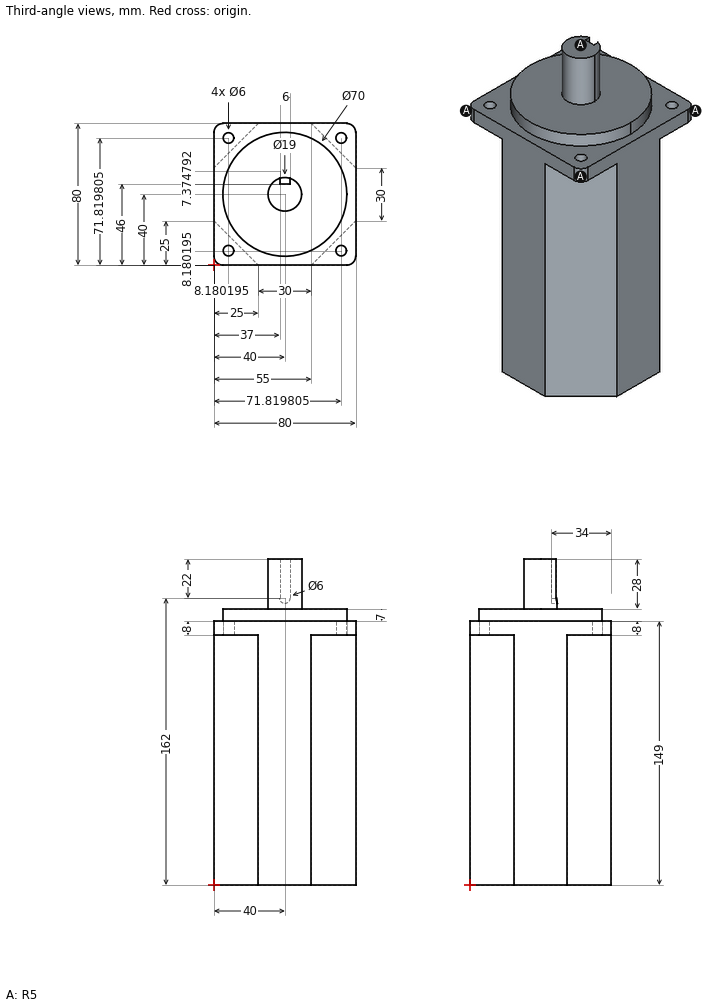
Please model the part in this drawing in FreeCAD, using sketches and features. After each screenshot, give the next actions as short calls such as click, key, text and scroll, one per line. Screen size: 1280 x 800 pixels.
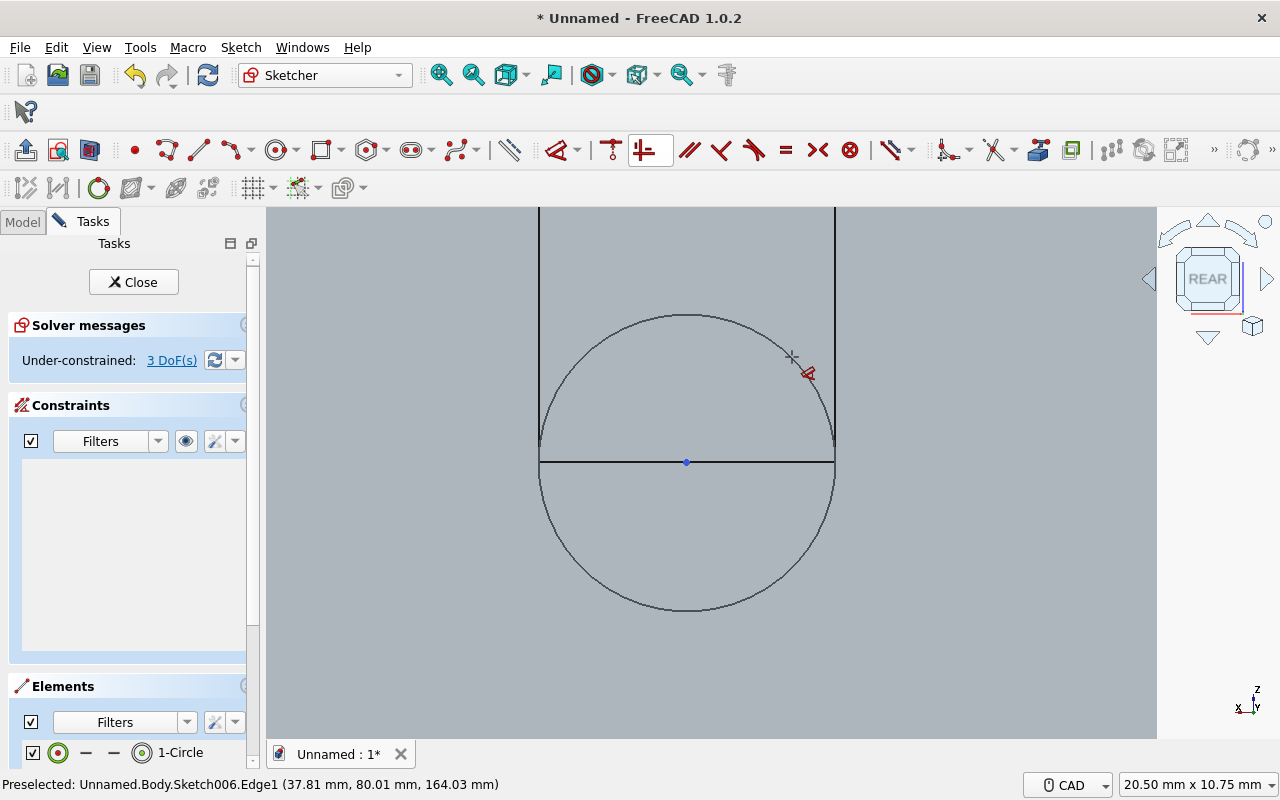
click(792, 358)
click(815, 335)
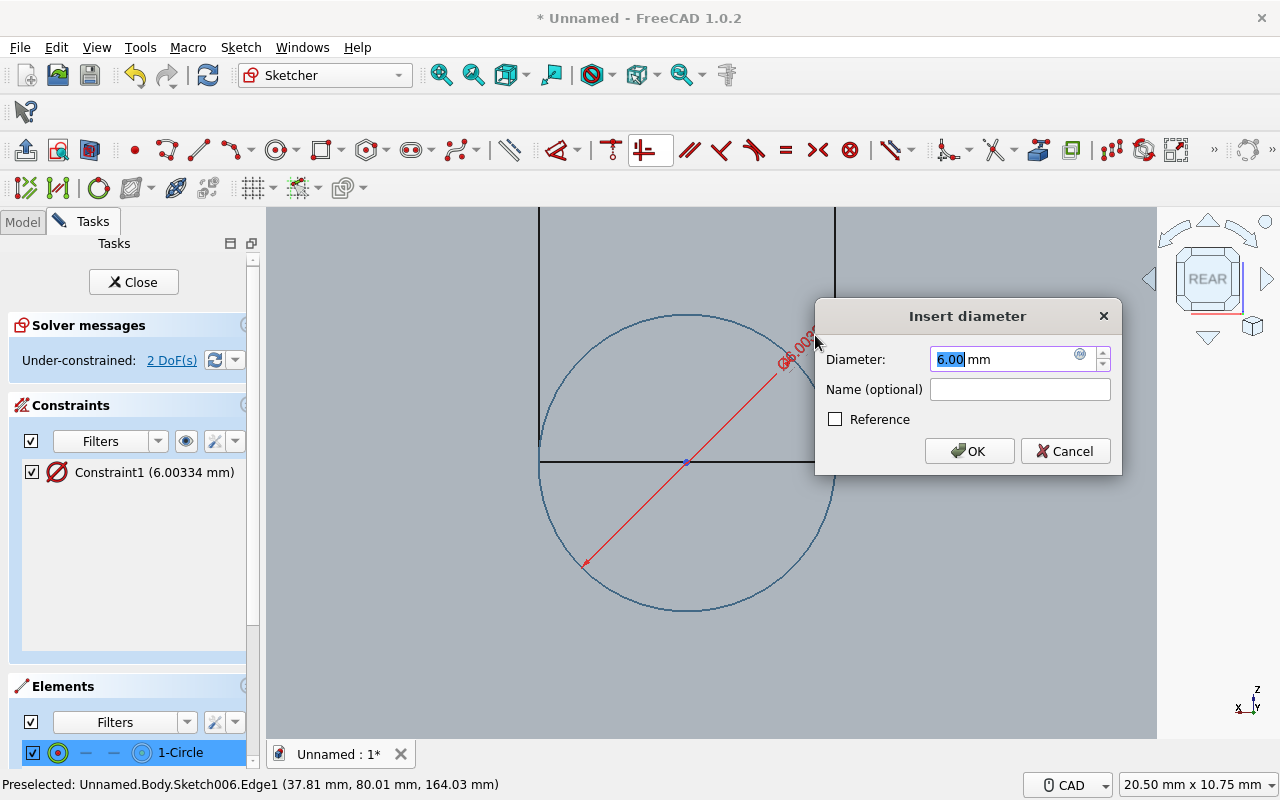
text(6)
key(Return)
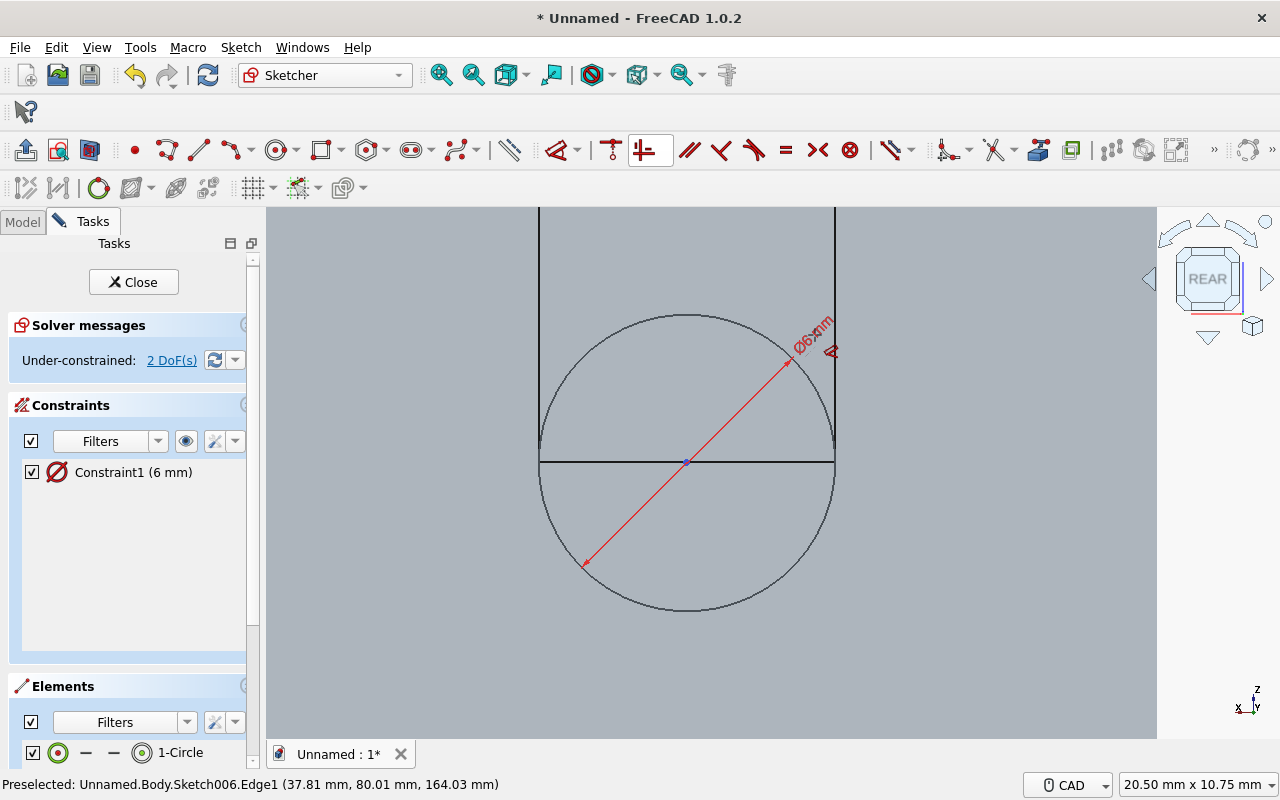
click(687, 463)
click(901, 429)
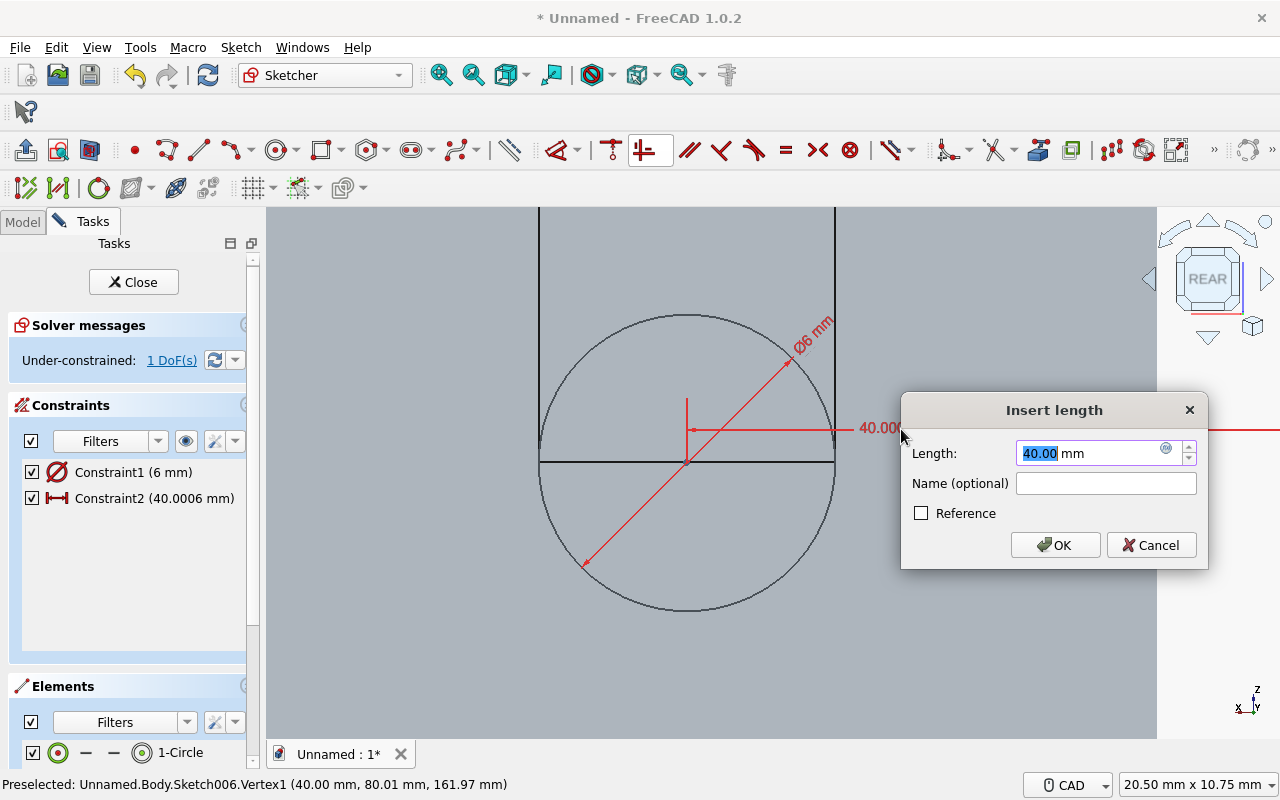
text(40)
key(Return)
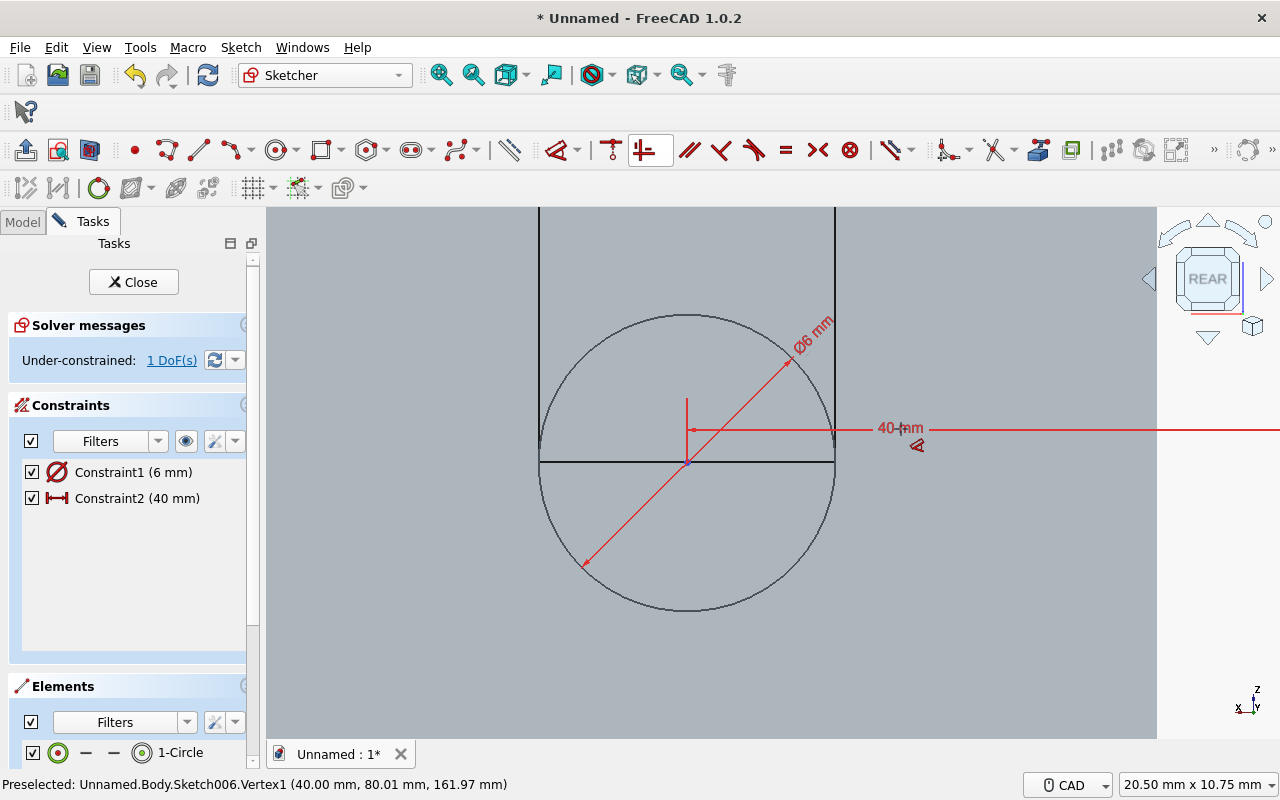
click(687, 463)
click(653, 587)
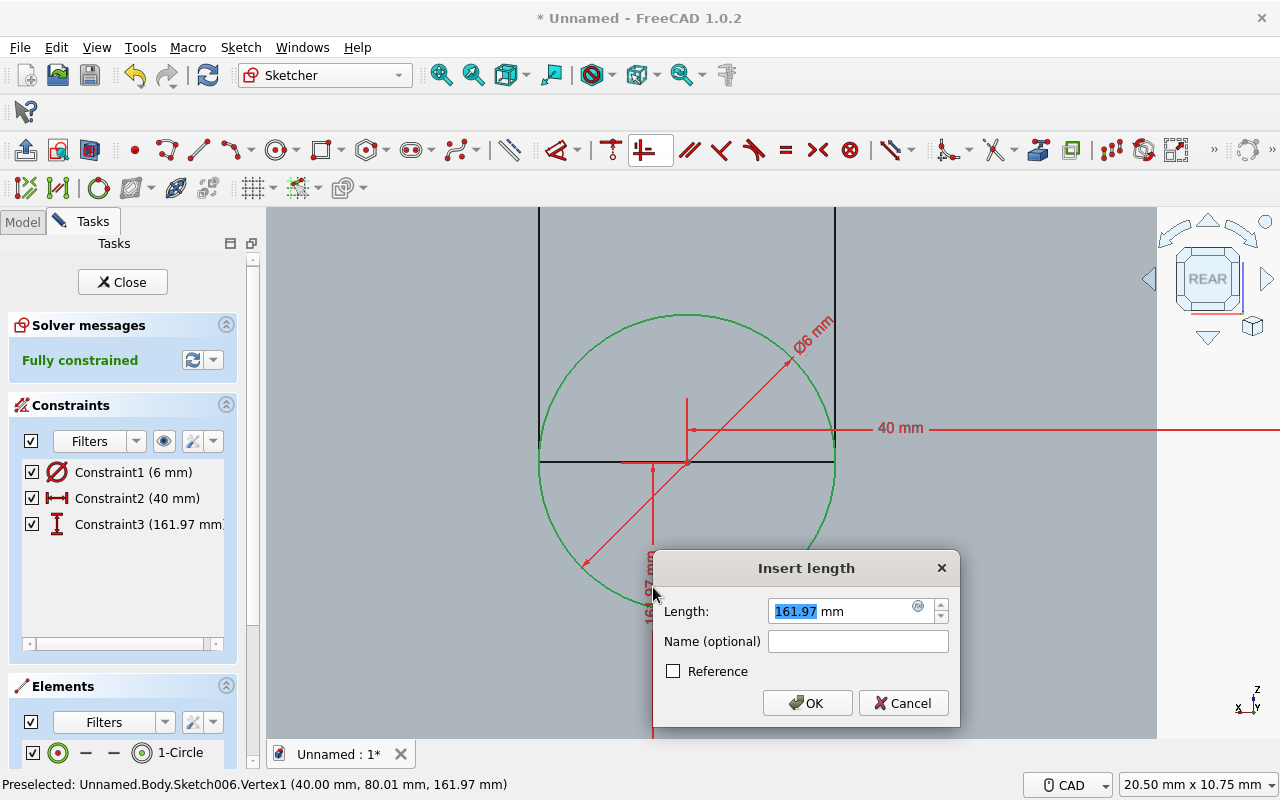
text(162)
key(Return)
key(Escape)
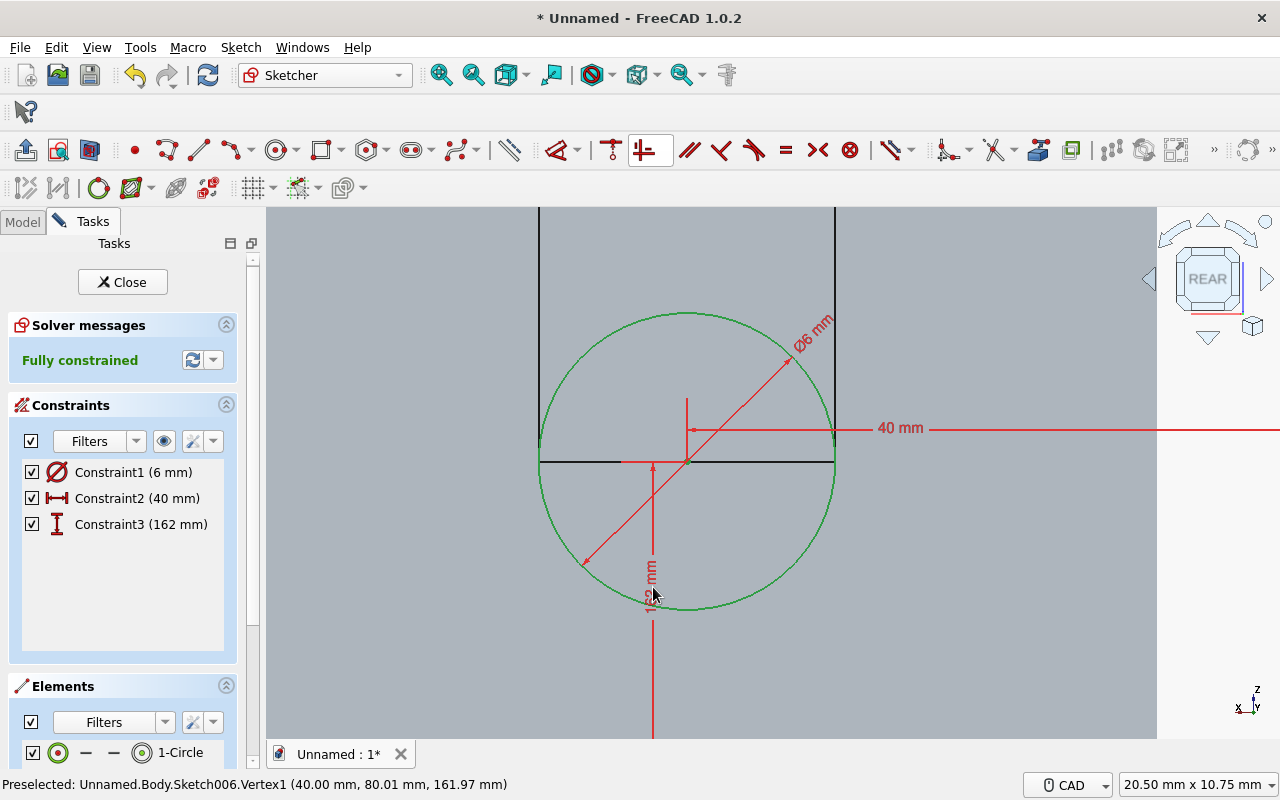
click(123, 282)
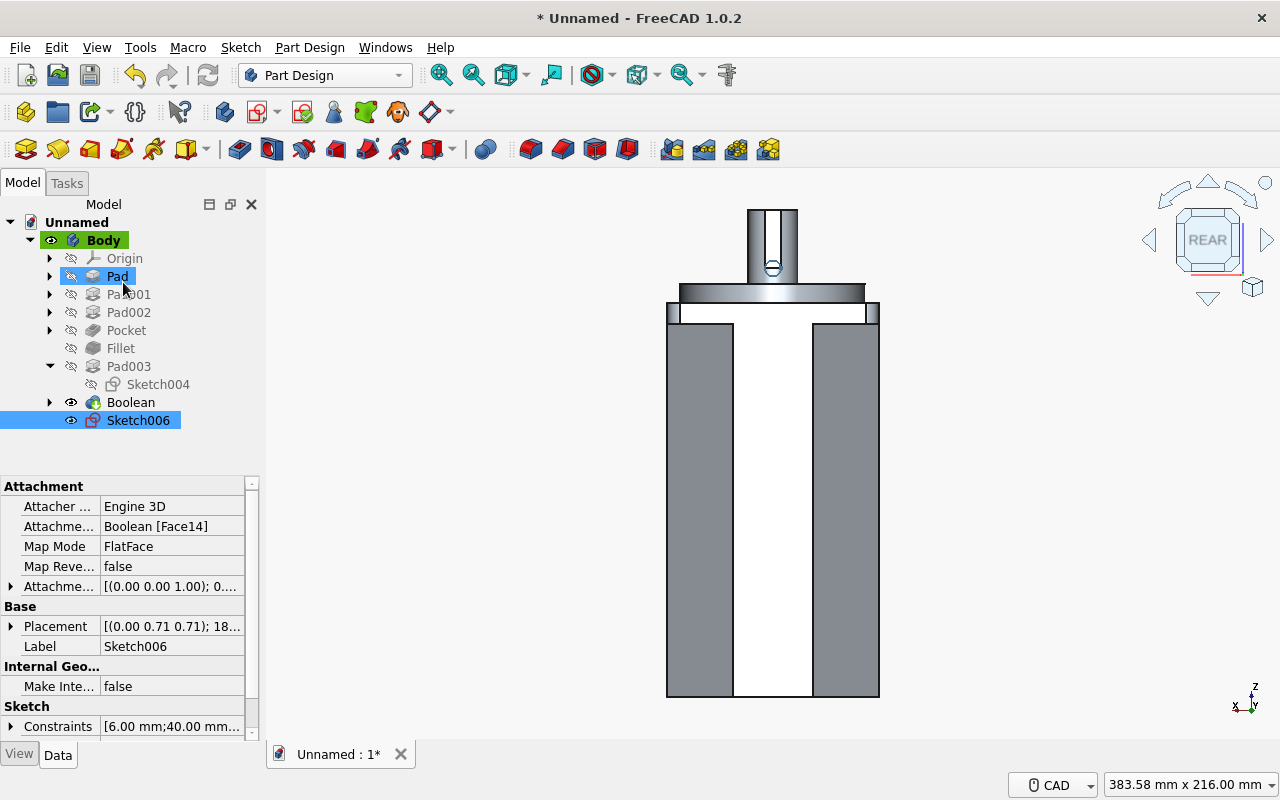
click(240, 150)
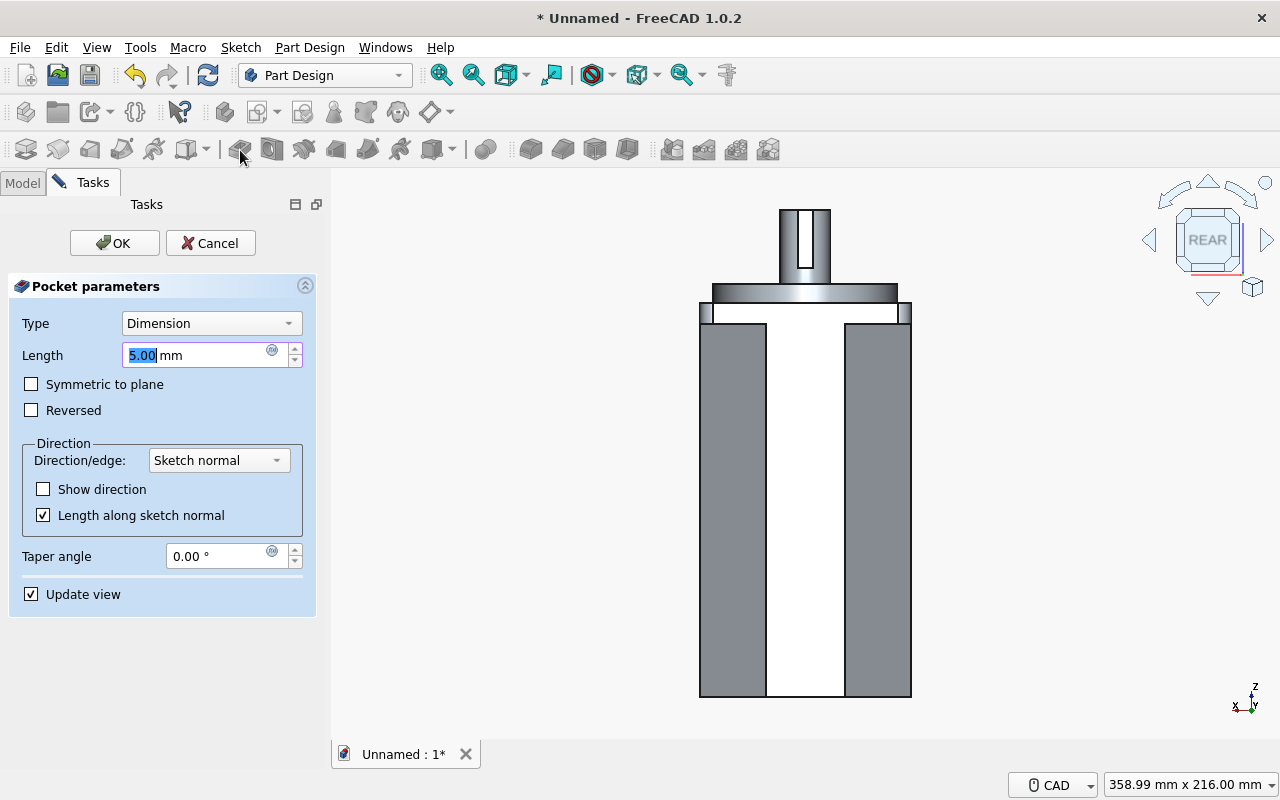
text(34)
key(Tab)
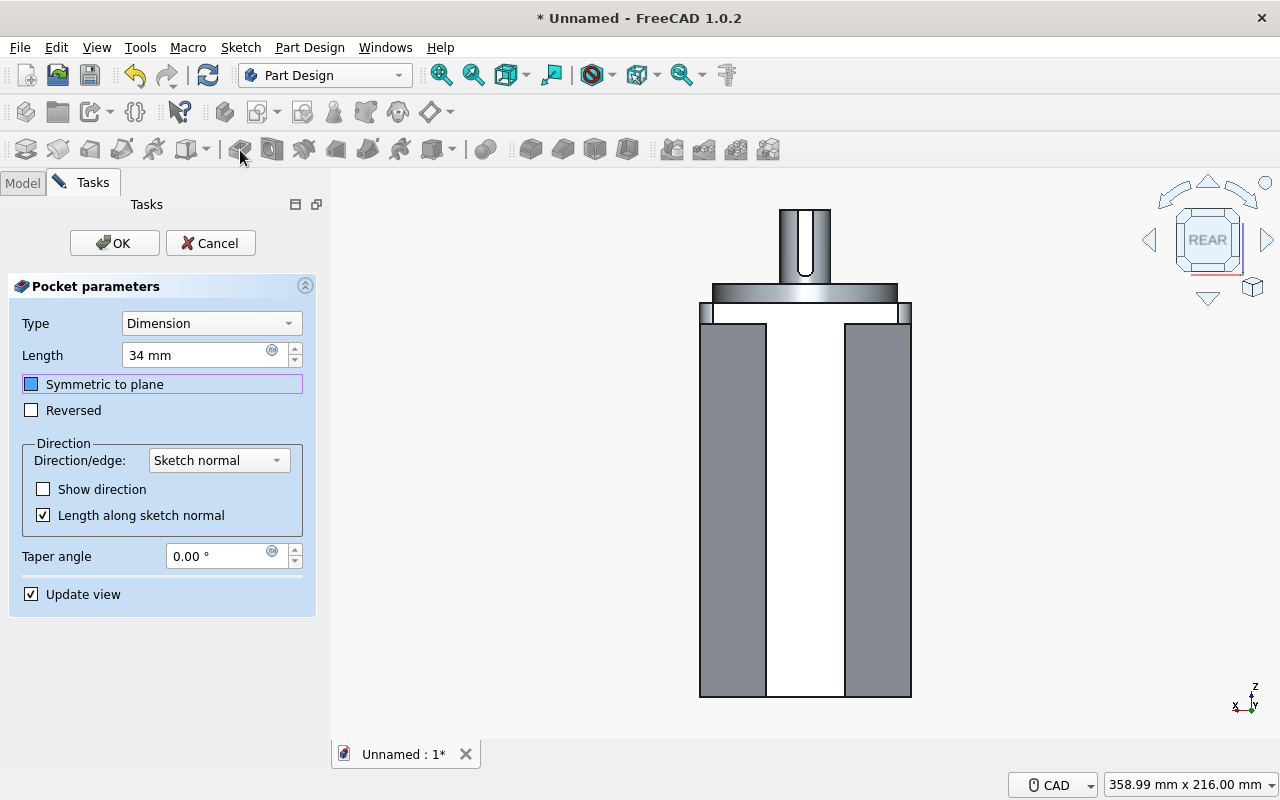
click(115, 243)